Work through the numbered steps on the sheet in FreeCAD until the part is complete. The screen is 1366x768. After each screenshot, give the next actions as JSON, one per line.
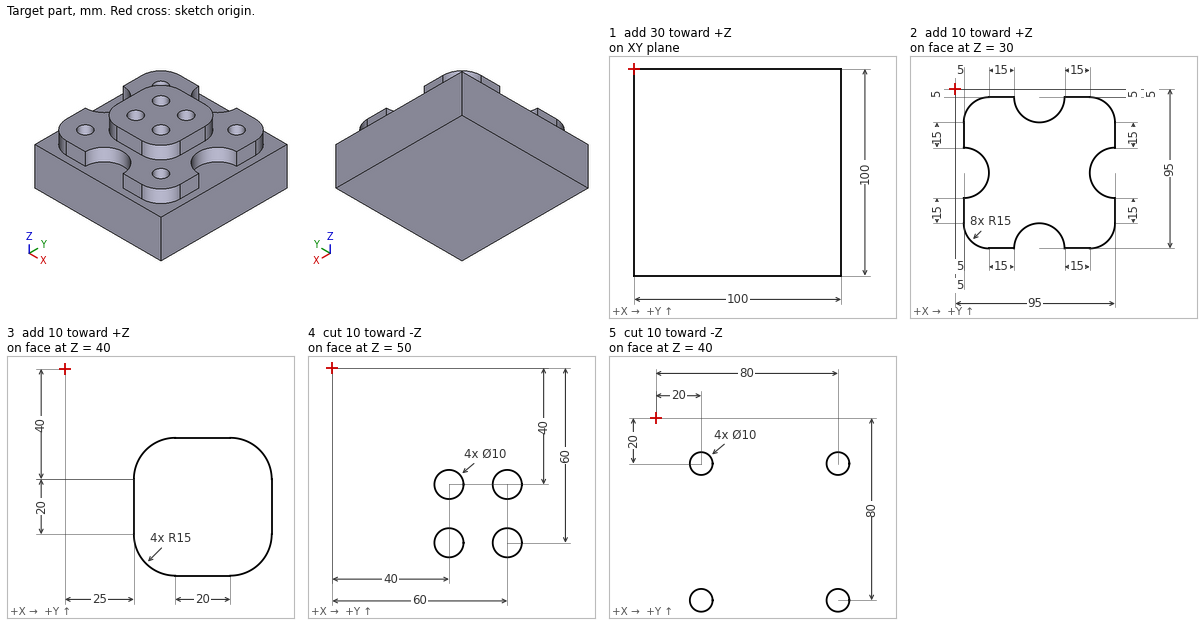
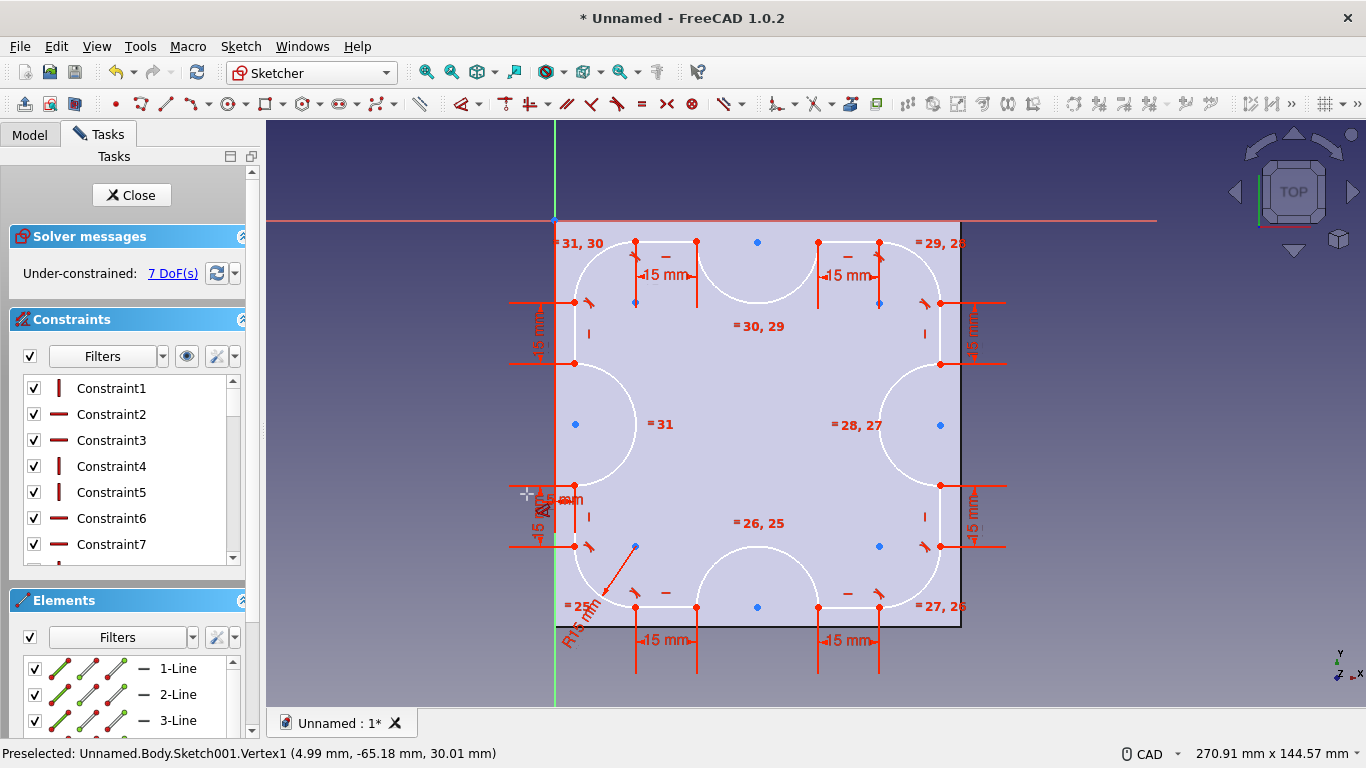
{"action": "scroll", "coordinate": [879, 242], "scroll_direction": "up", "scroll_amount": 4}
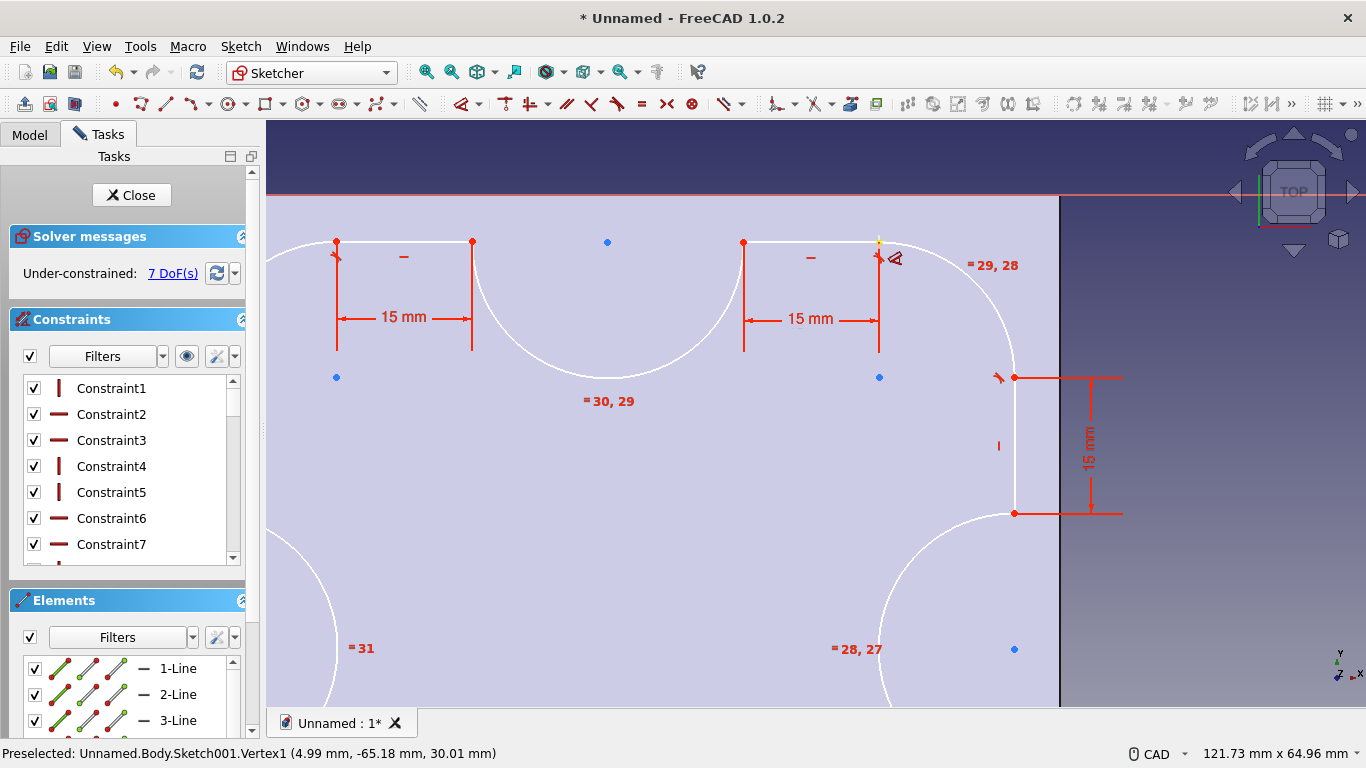
{"action": "left_click", "coordinate": [879, 242]}
{"action": "left_click", "coordinate": [913, 219]}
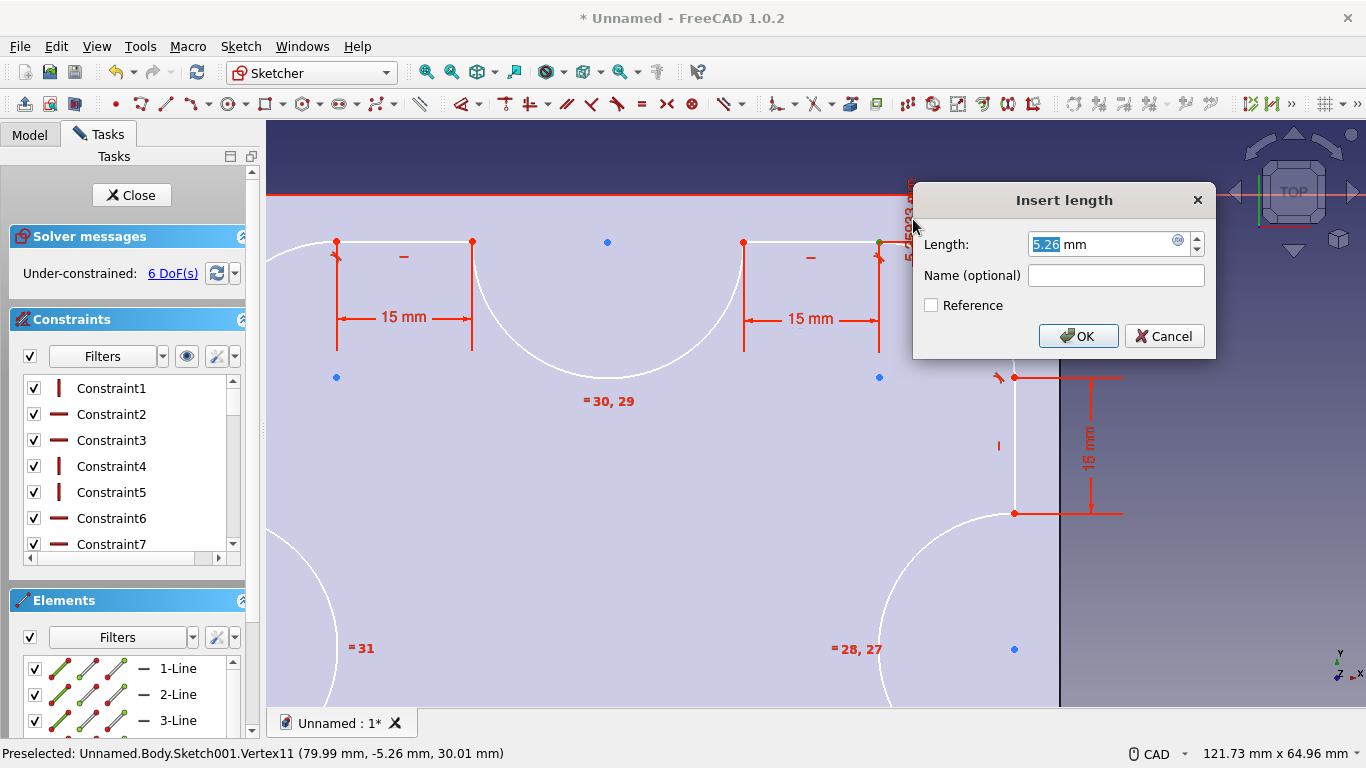
{"action": "type", "text": "5"}
{"action": "key", "text": "Return"}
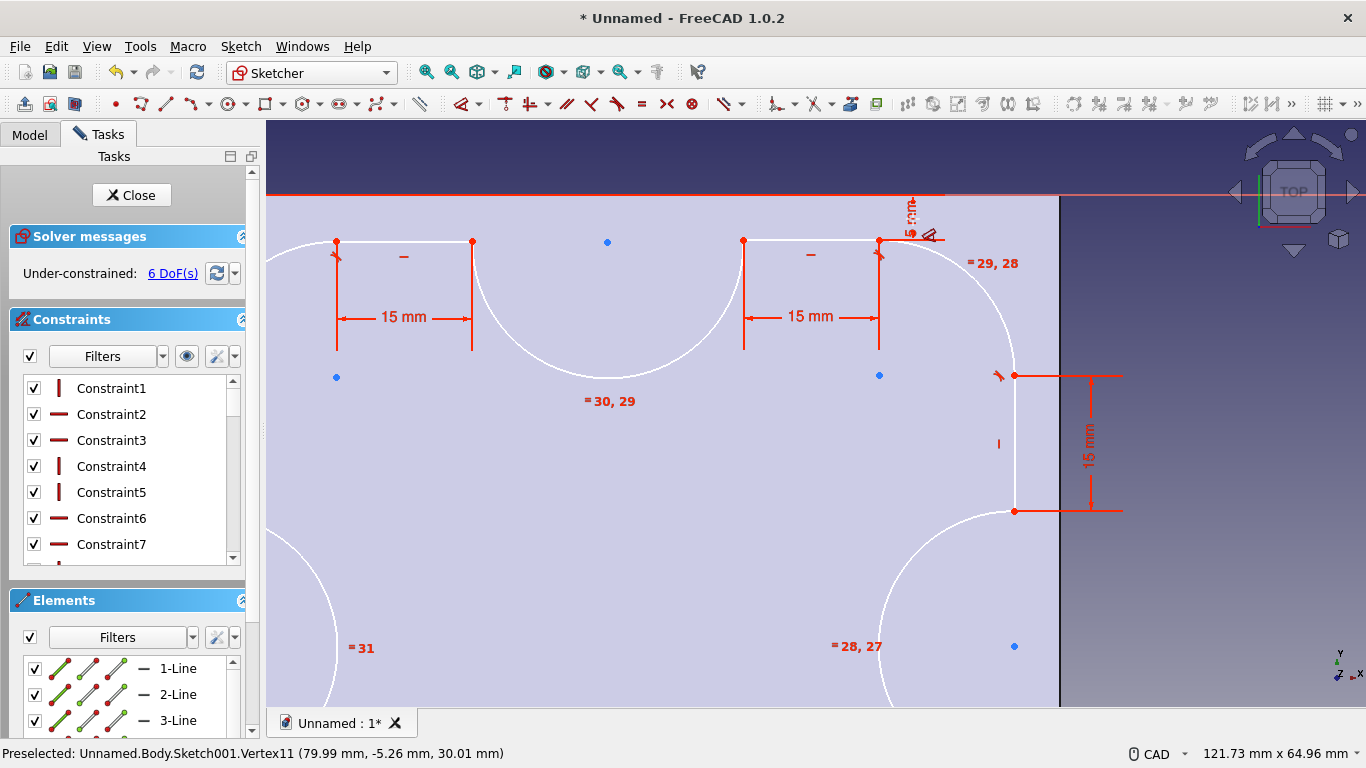
{"action": "left_click", "coordinate": [472, 242]}
{"action": "left_click", "coordinate": [506, 218]}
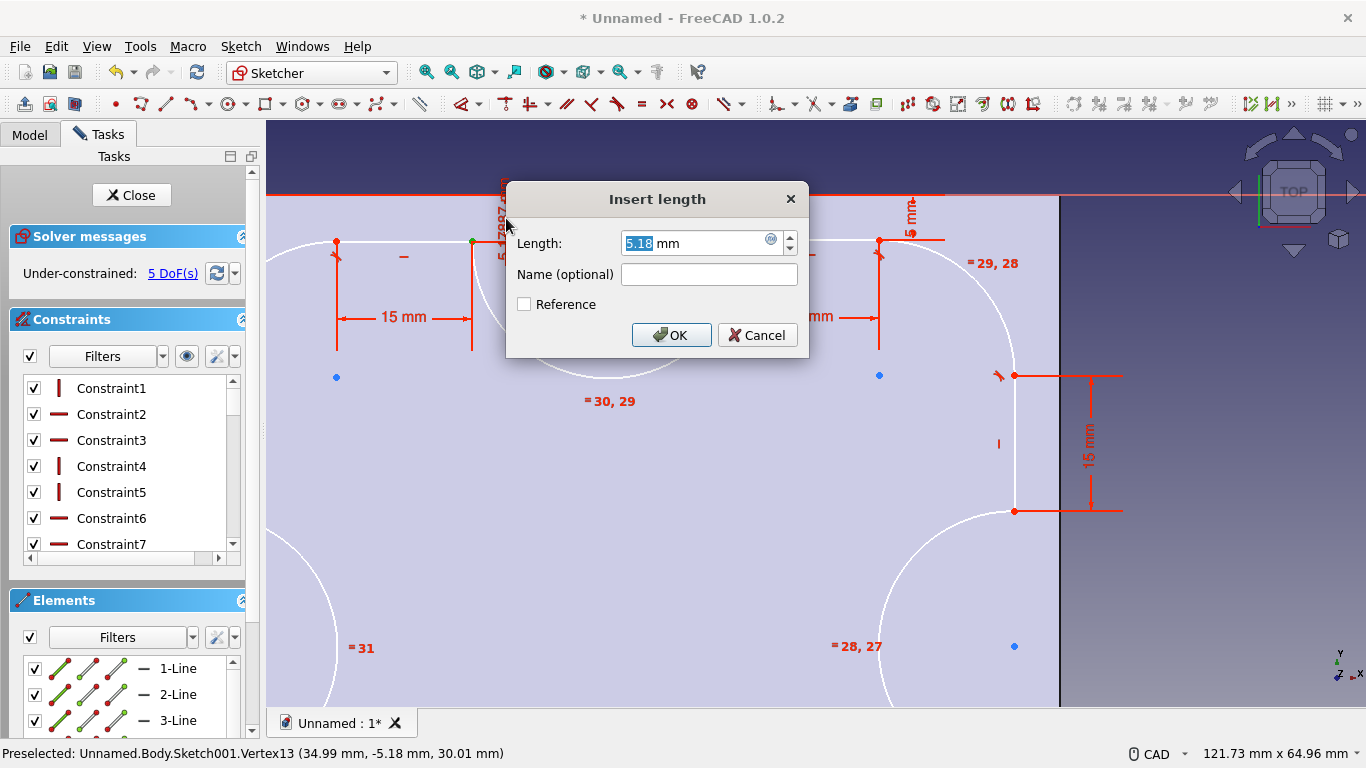
{"action": "type", "text": "5"}
{"action": "key", "text": "Return"}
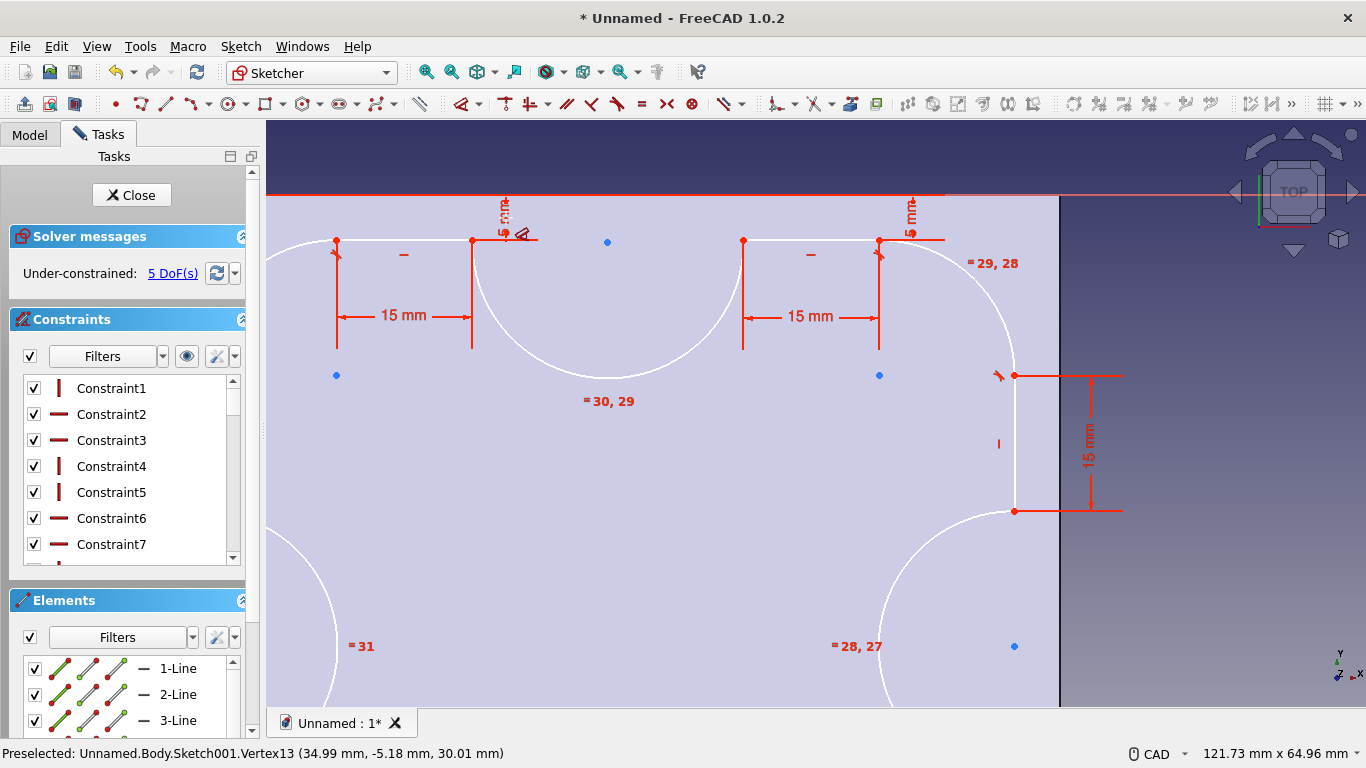
{"action": "scroll", "coordinate": [880, 242], "scroll_direction": "down", "scroll_amount": 4}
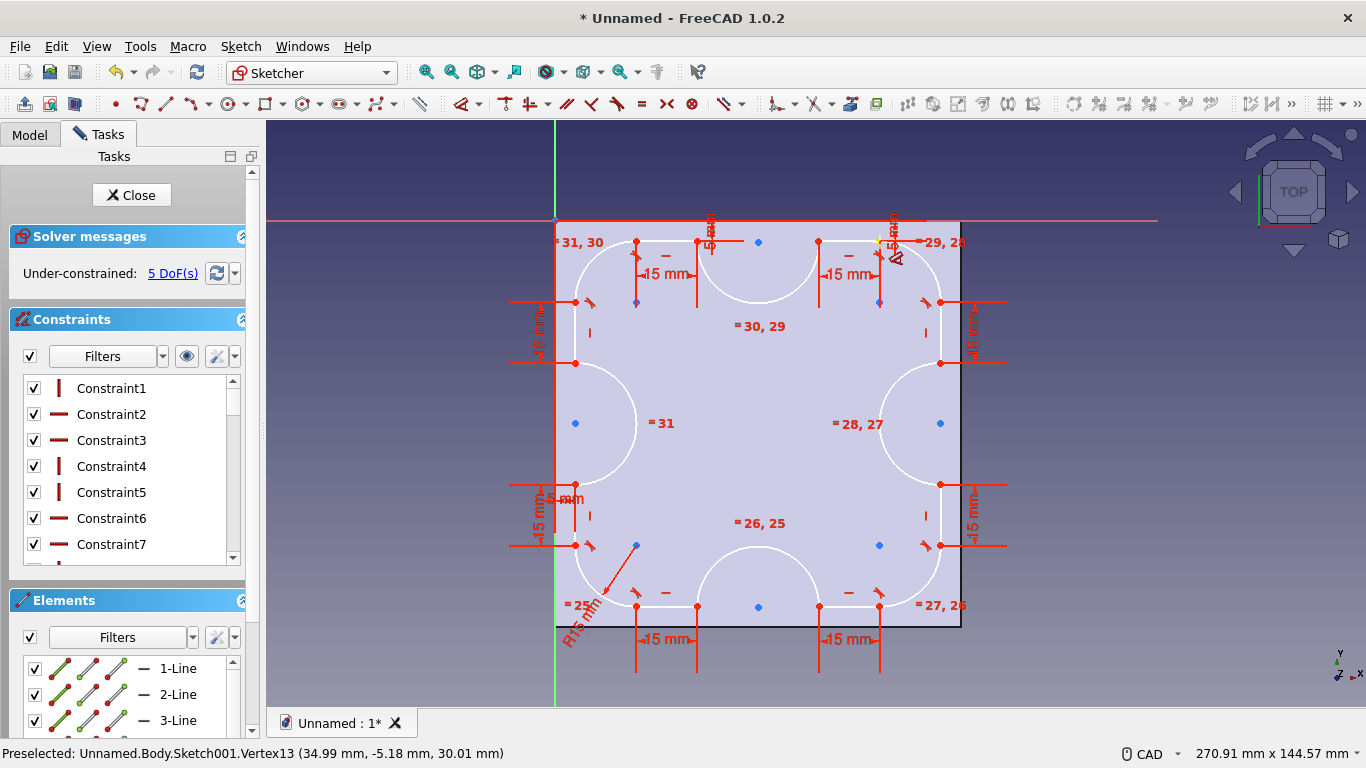
{"action": "scroll", "coordinate": [575, 302], "scroll_direction": "up", "scroll_amount": 4}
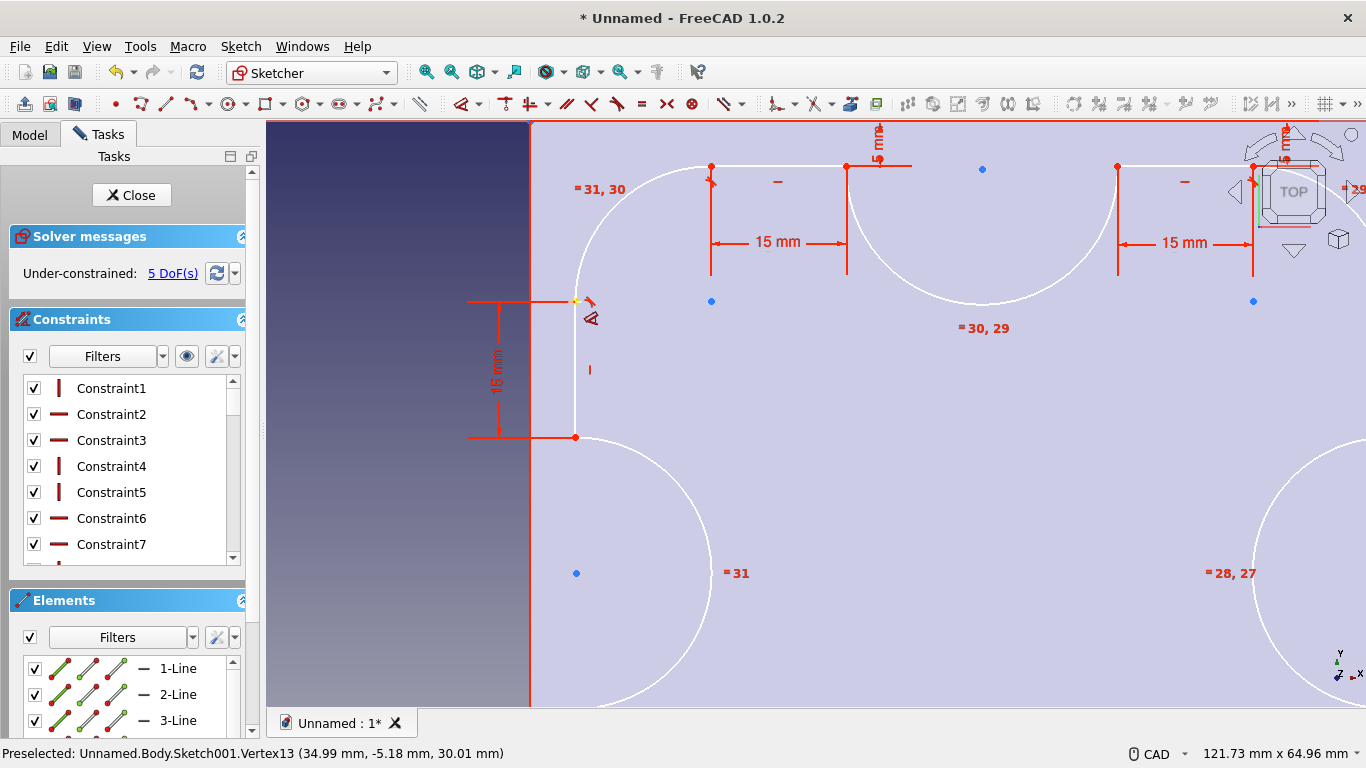
{"action": "left_click", "coordinate": [575, 302]}
{"action": "left_click", "coordinate": [553, 336]}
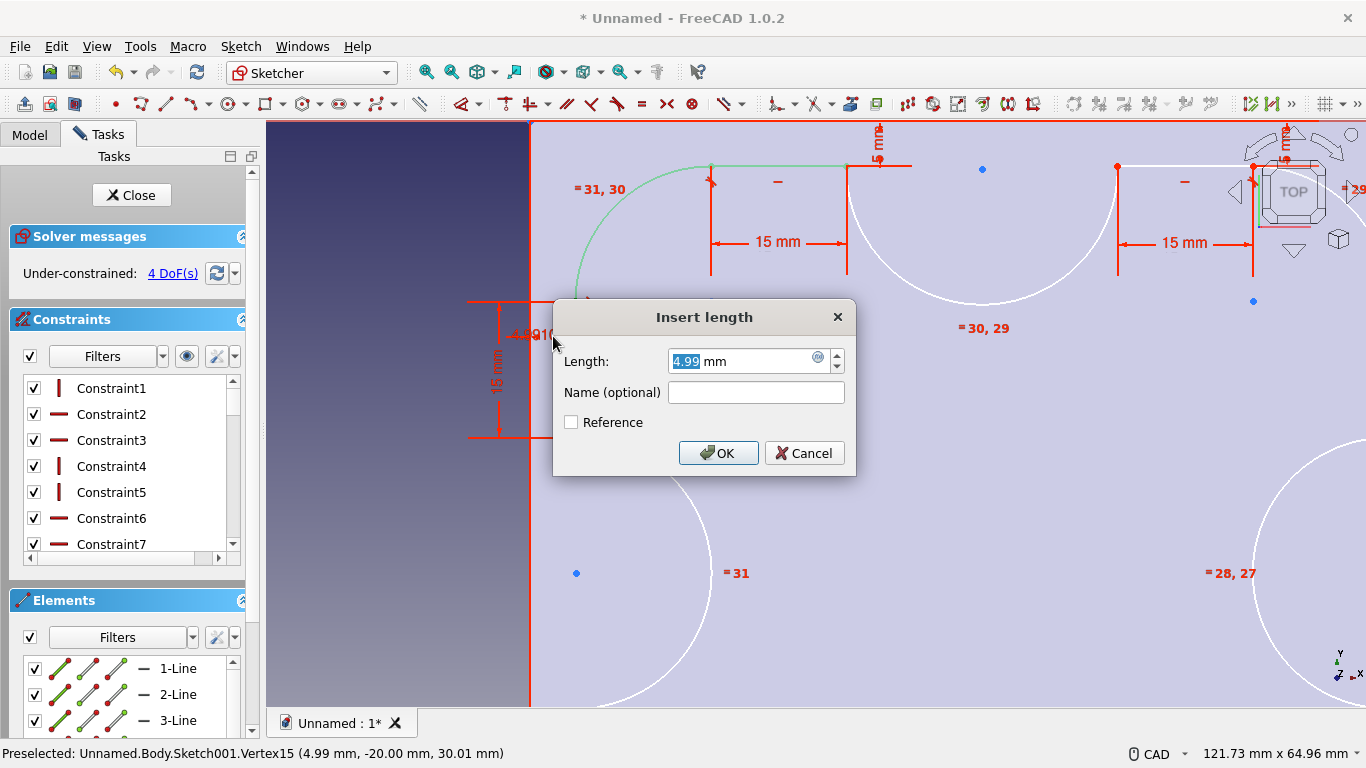
{"action": "type", "text": "5"}
{"action": "key", "text": "Return"}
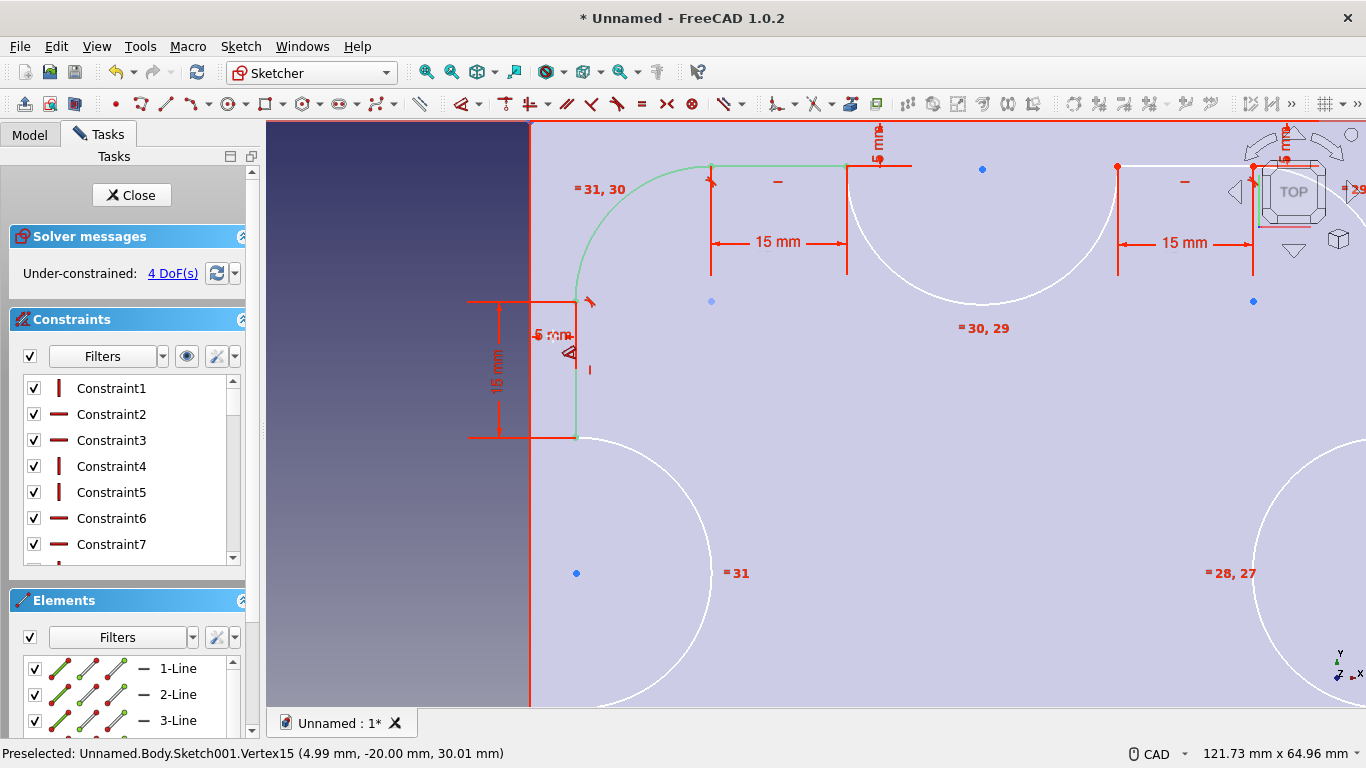
{"action": "left_click", "coordinate": [982, 169]}
{"action": "left_click", "coordinate": [496, 159]}